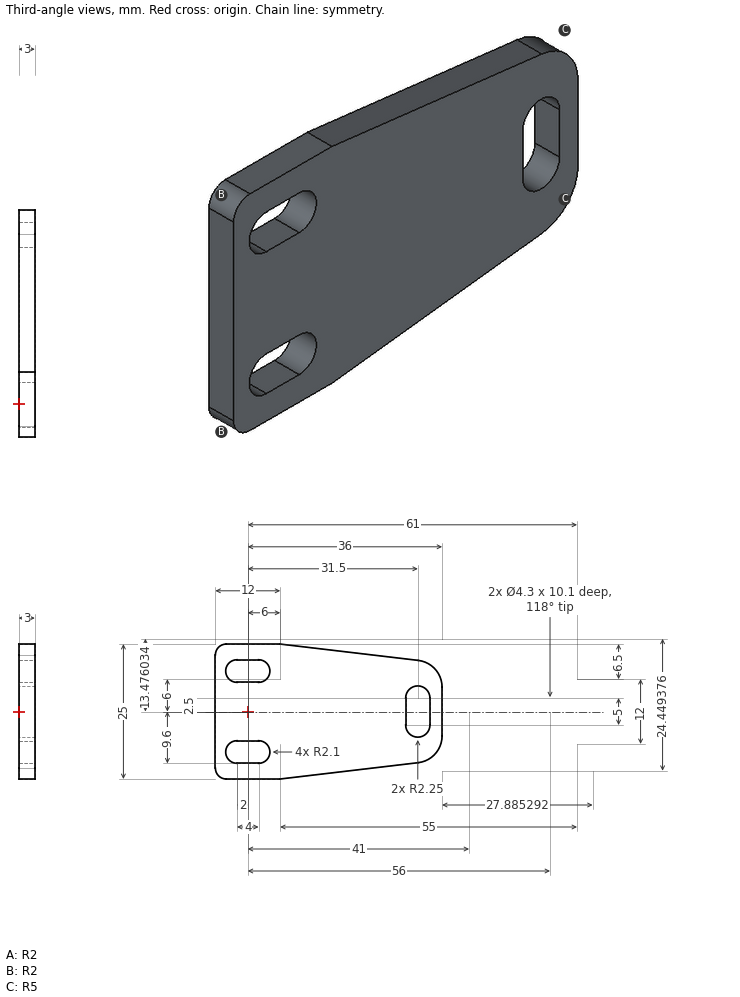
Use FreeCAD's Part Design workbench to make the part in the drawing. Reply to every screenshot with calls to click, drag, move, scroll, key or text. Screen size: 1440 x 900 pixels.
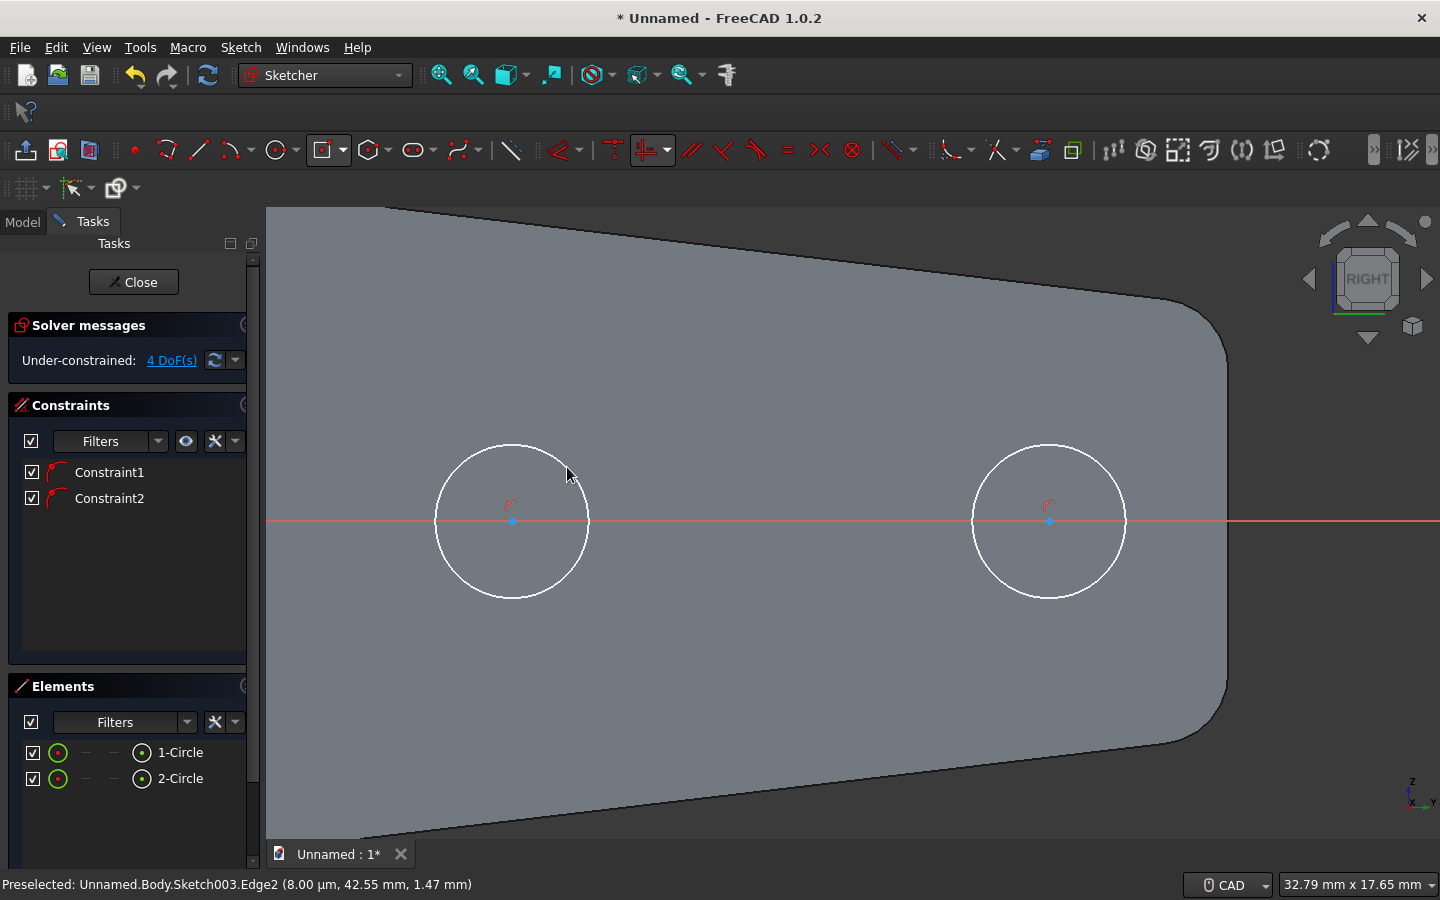
click(1103, 467)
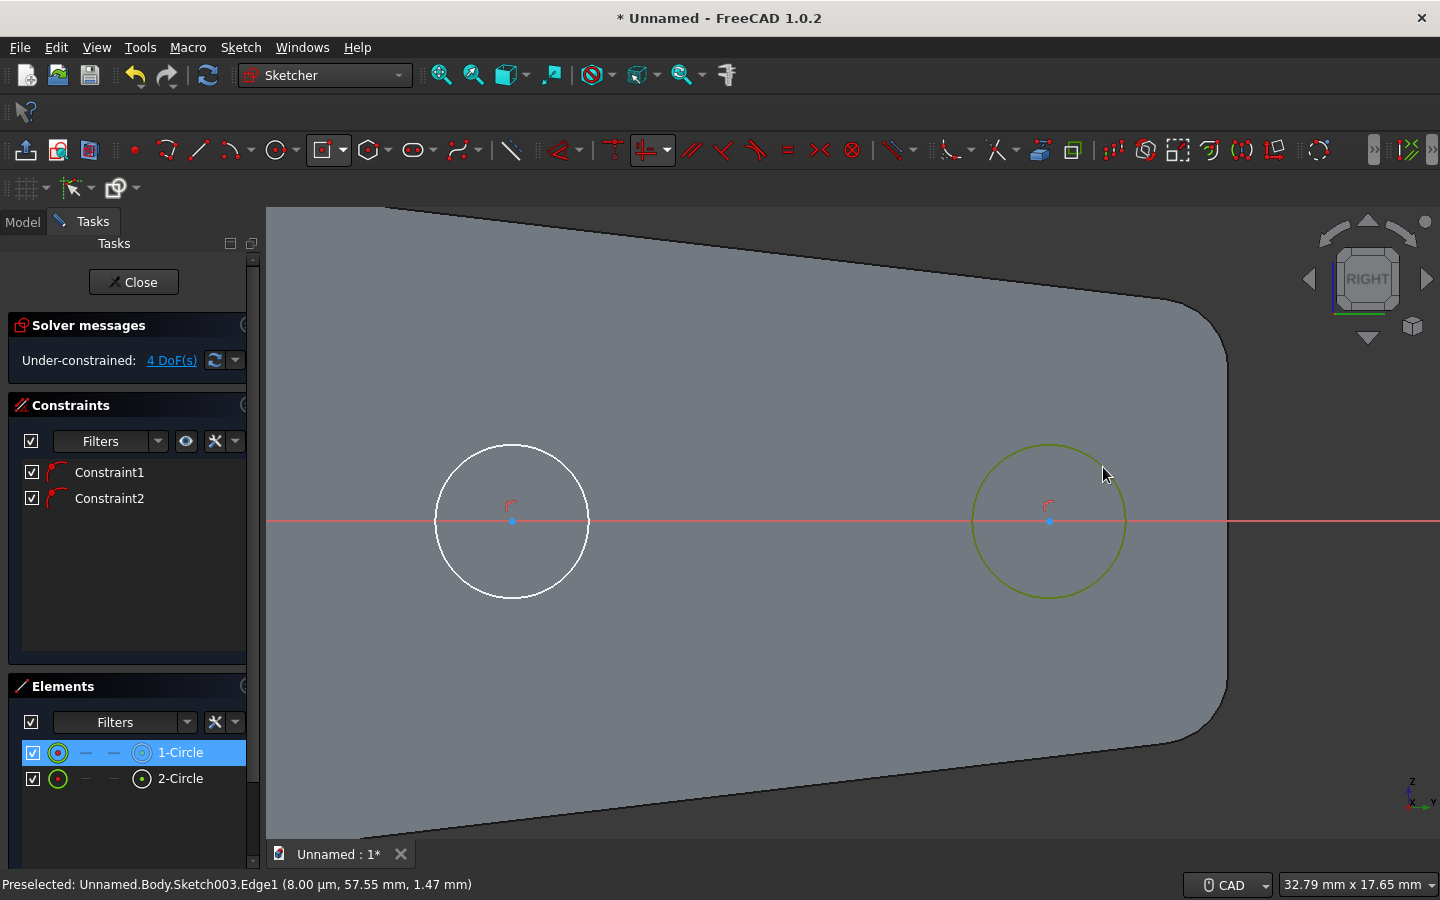
click(566, 467)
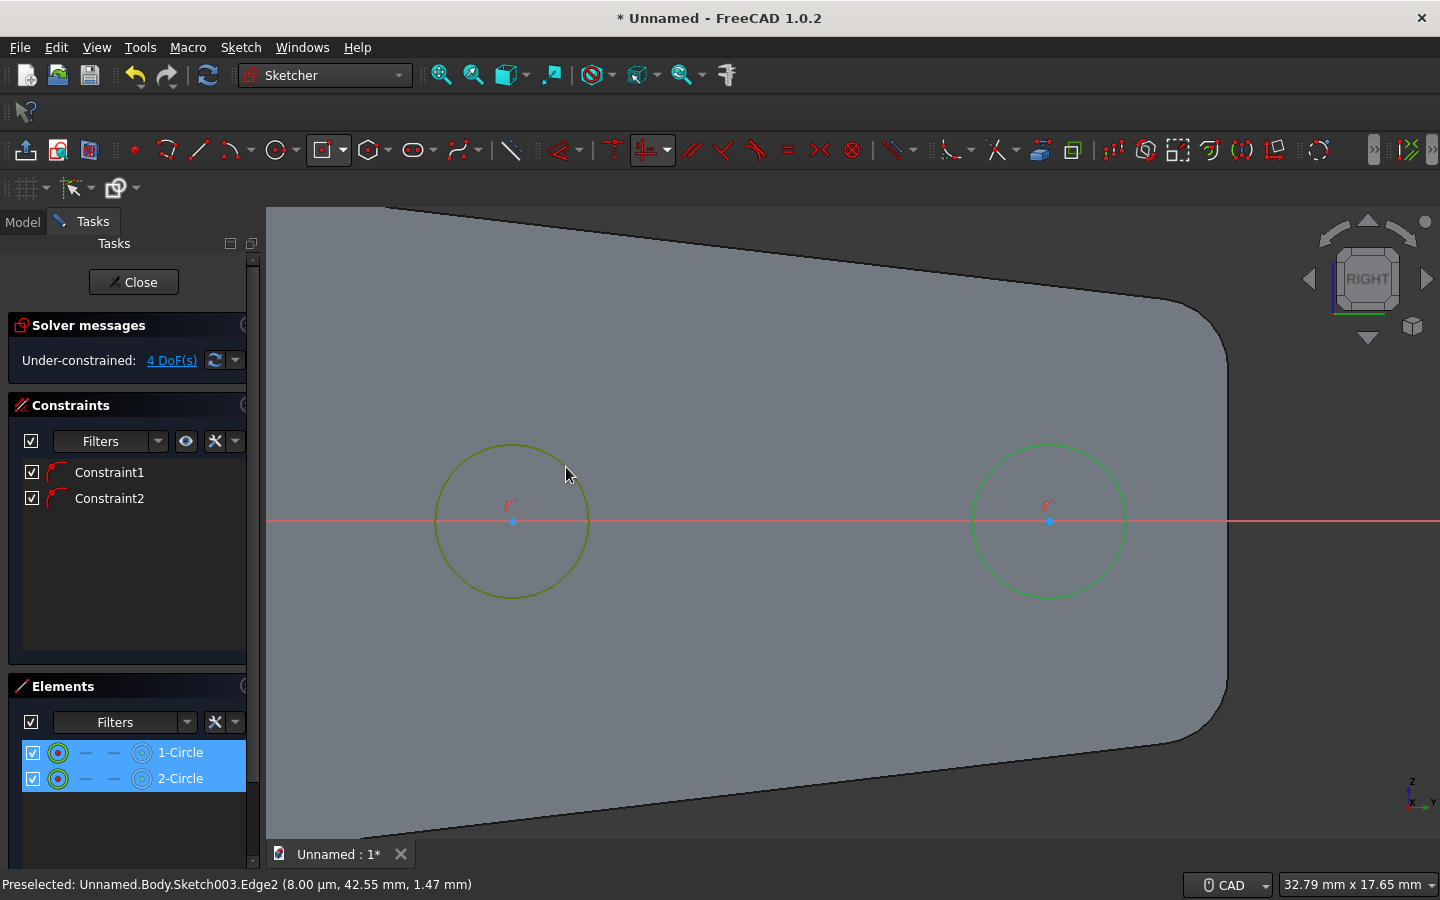
key(e)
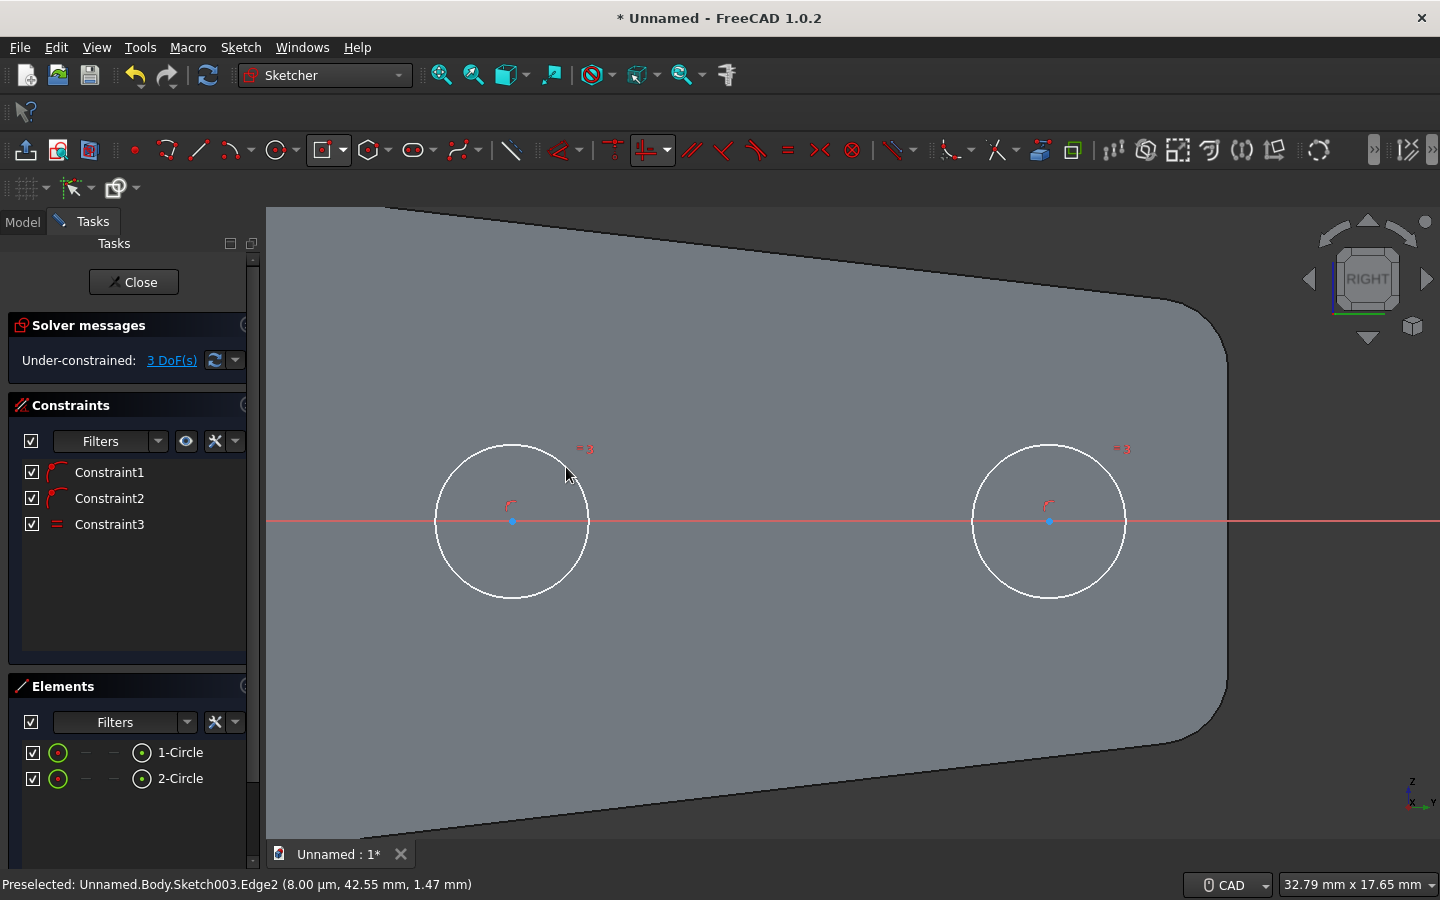
click(558, 150)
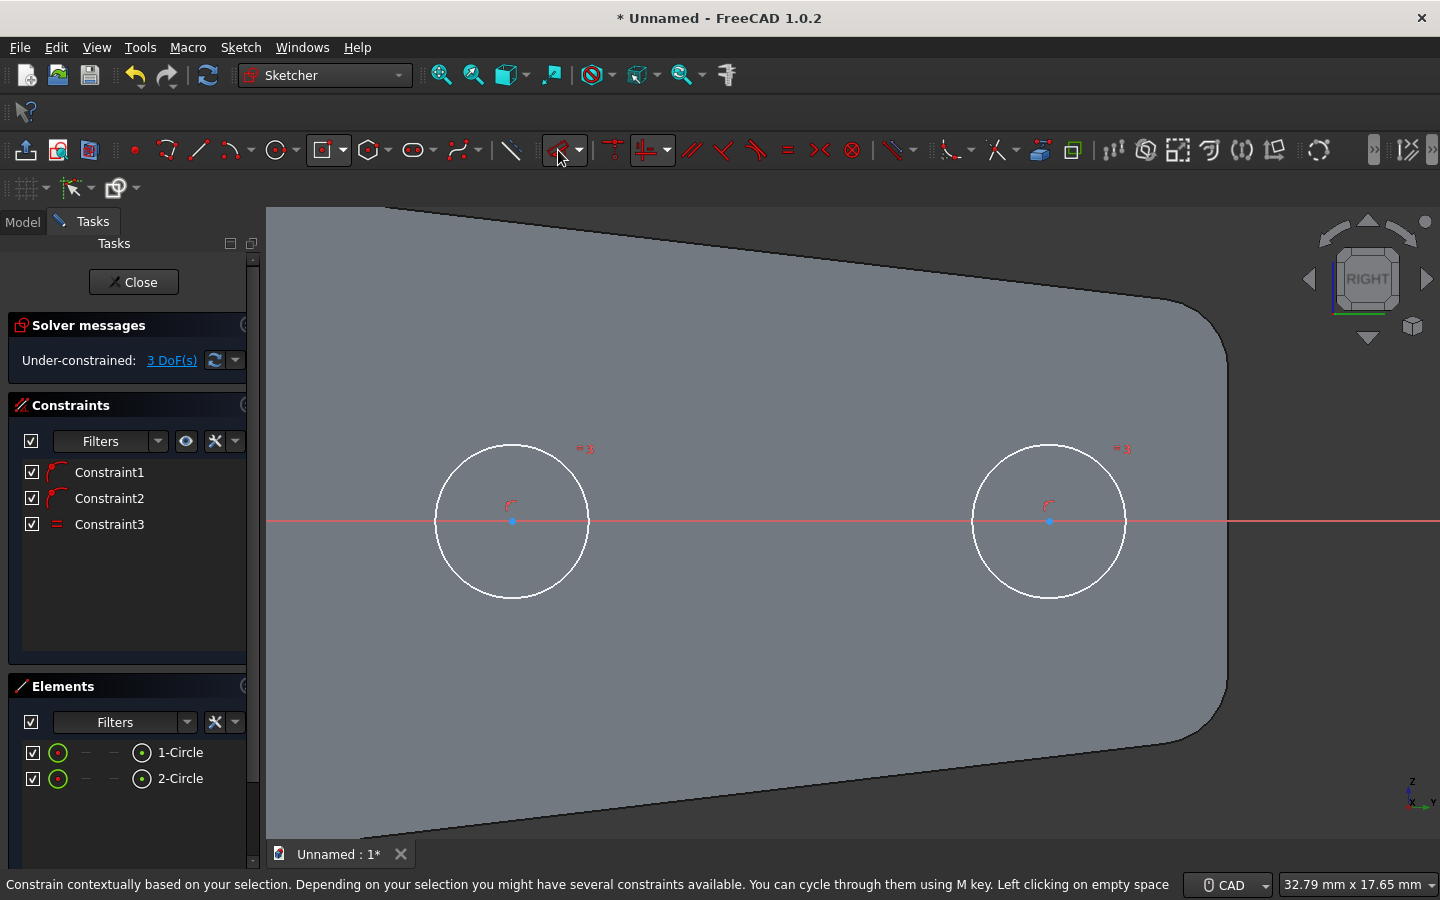
click(1103, 467)
click(1126, 444)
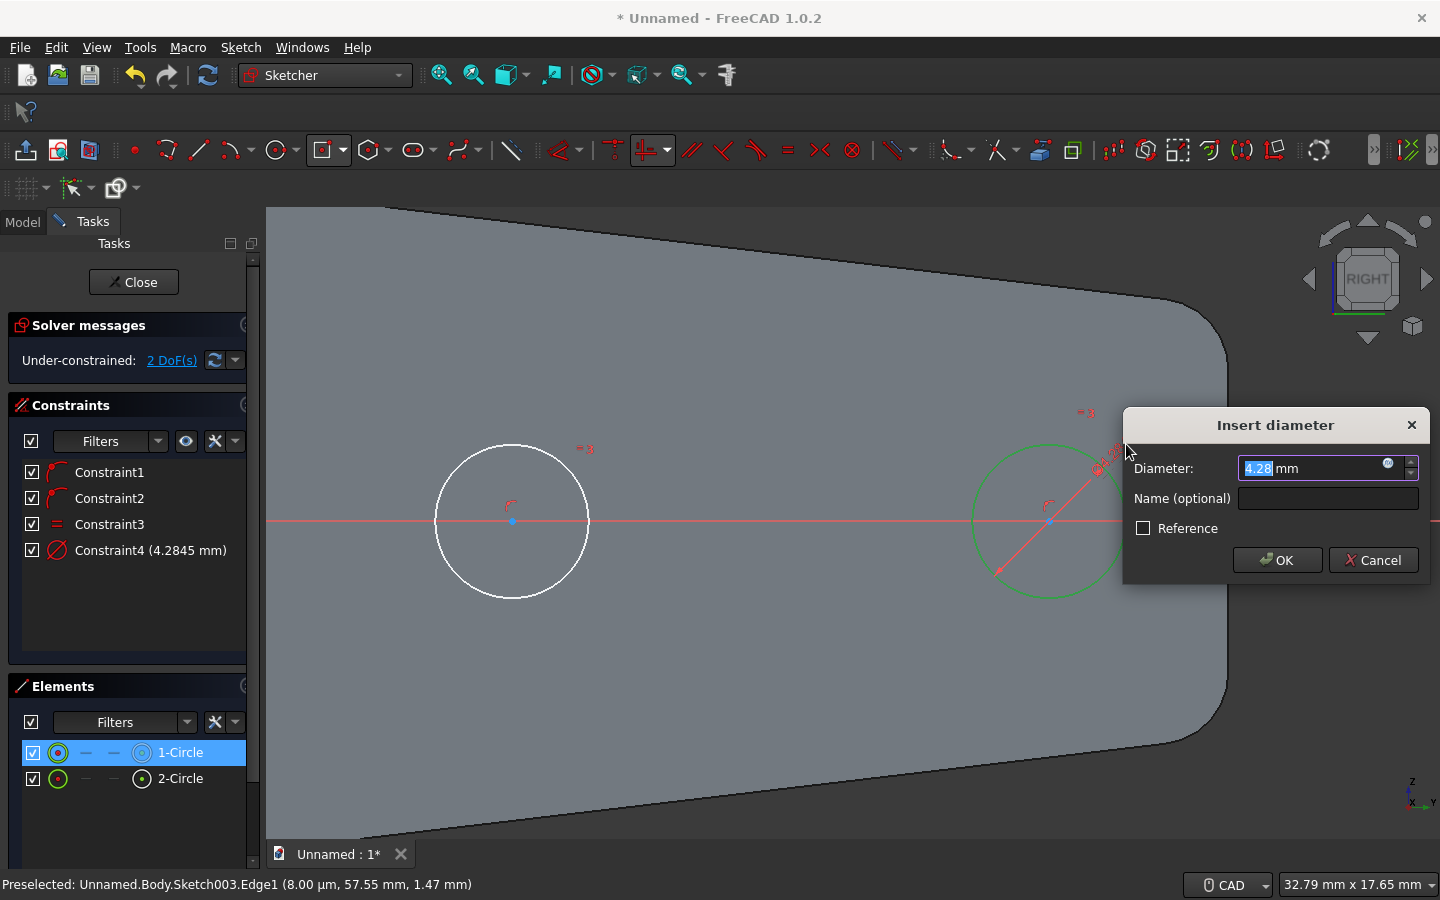
text(4.3)
key(Return)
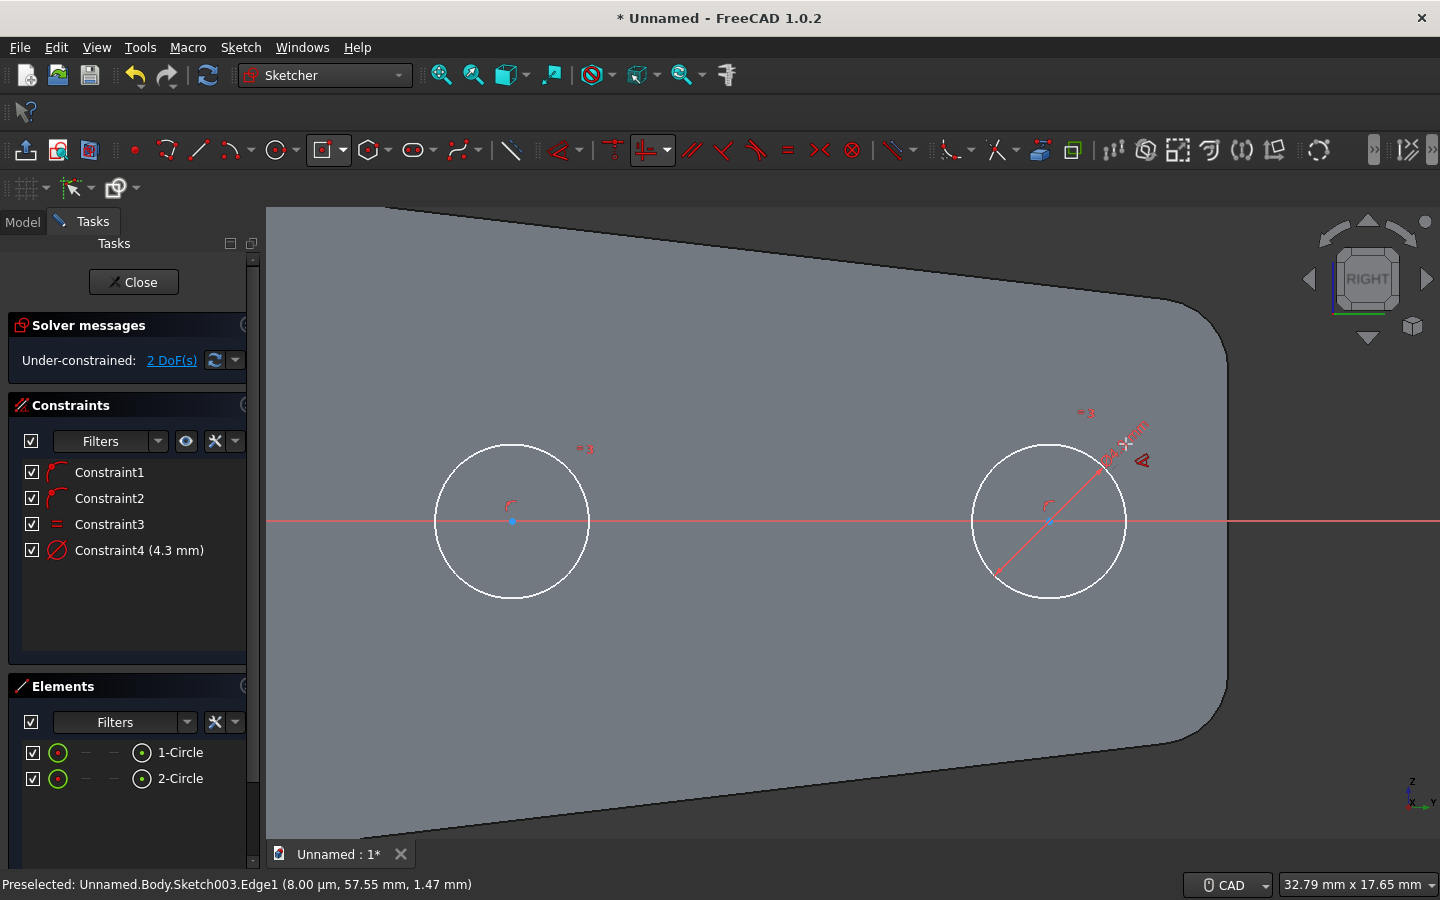
click(1049, 521)
click(672, 555)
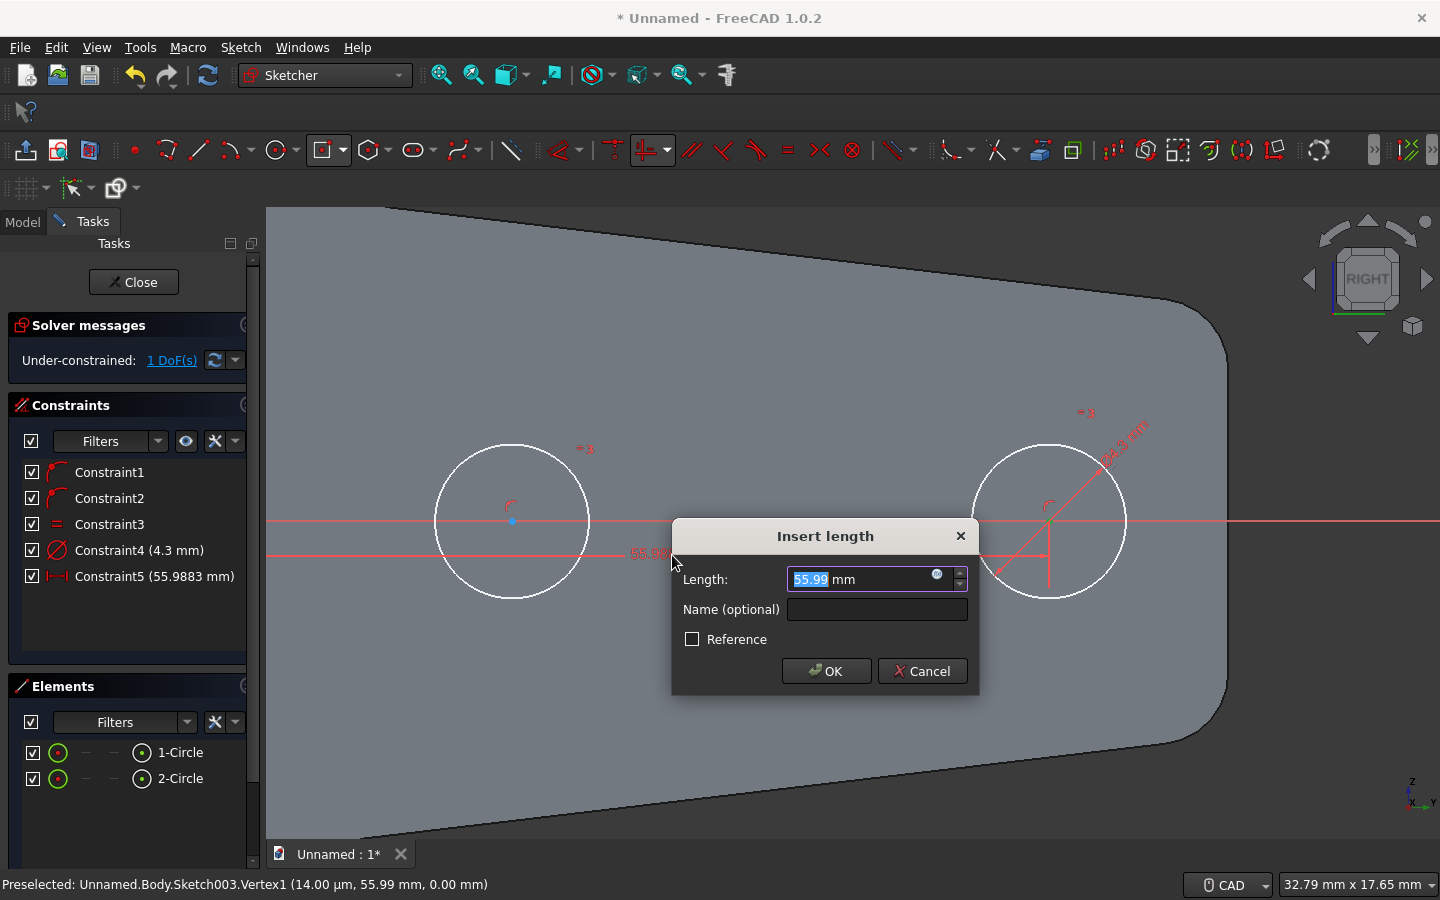
text(56)
key(Return)